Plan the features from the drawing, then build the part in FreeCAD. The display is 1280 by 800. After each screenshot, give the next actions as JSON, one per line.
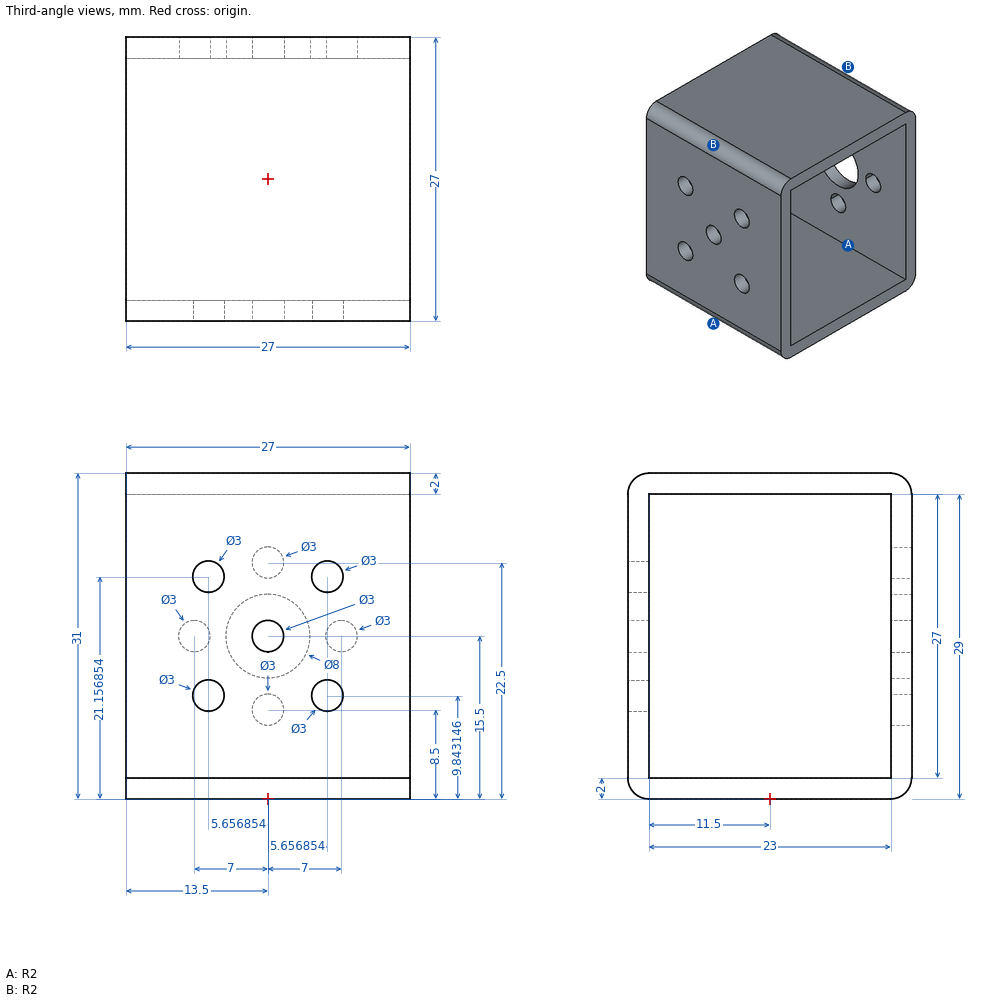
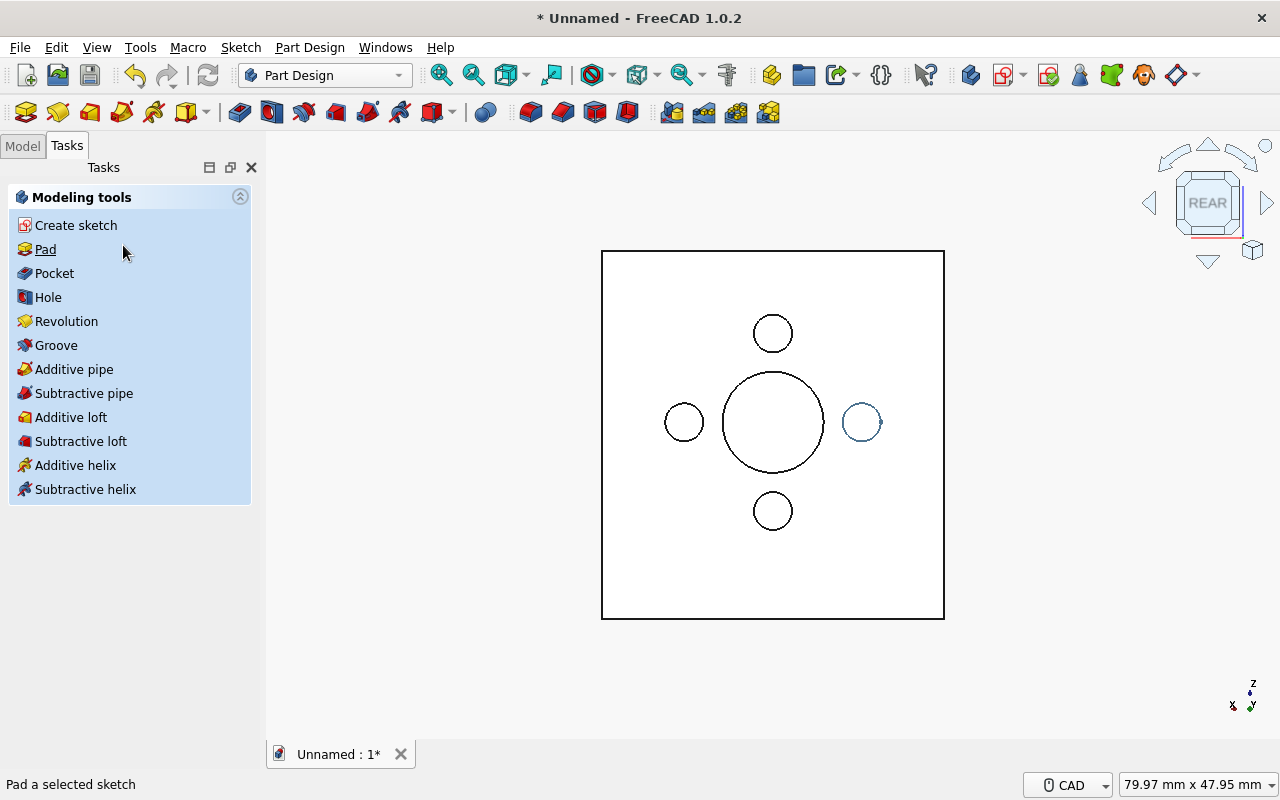
{"action": "left_click", "coordinate": [240, 112]}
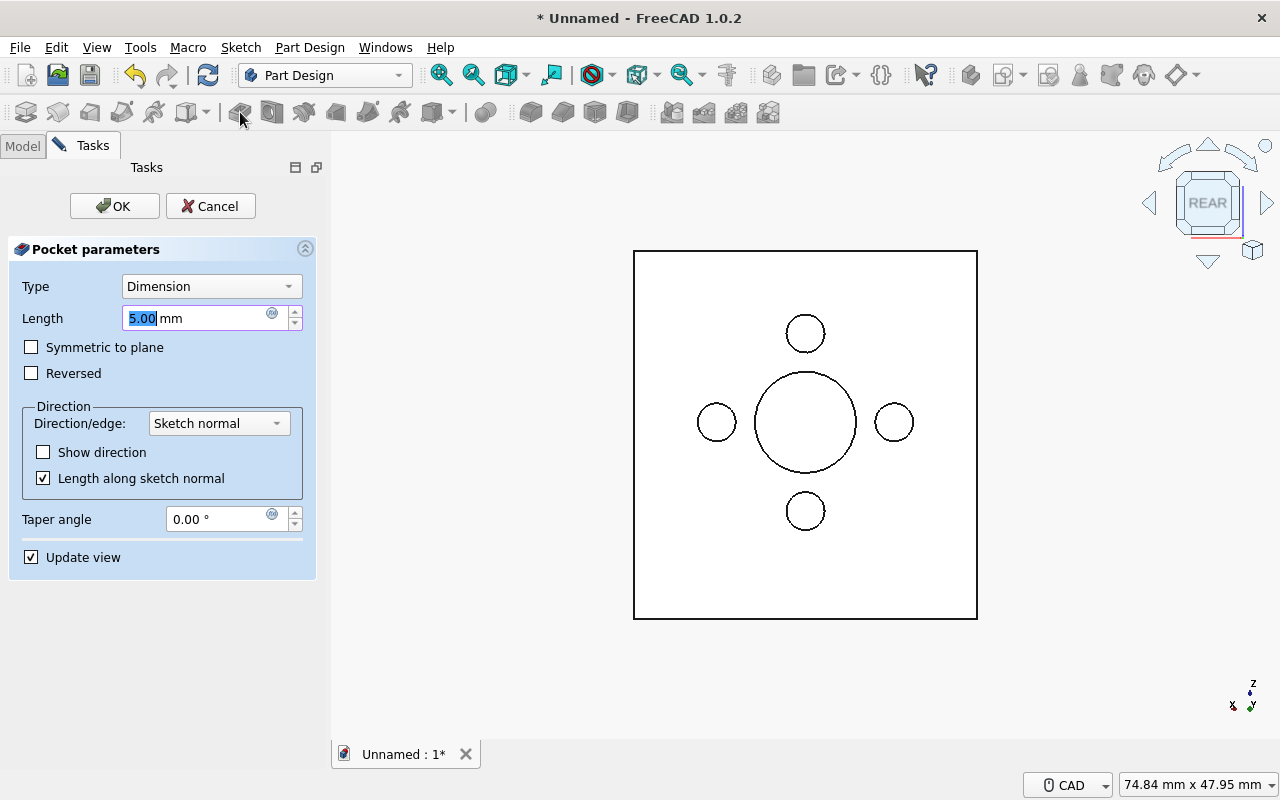
{"action": "left_click", "coordinate": [212, 286]}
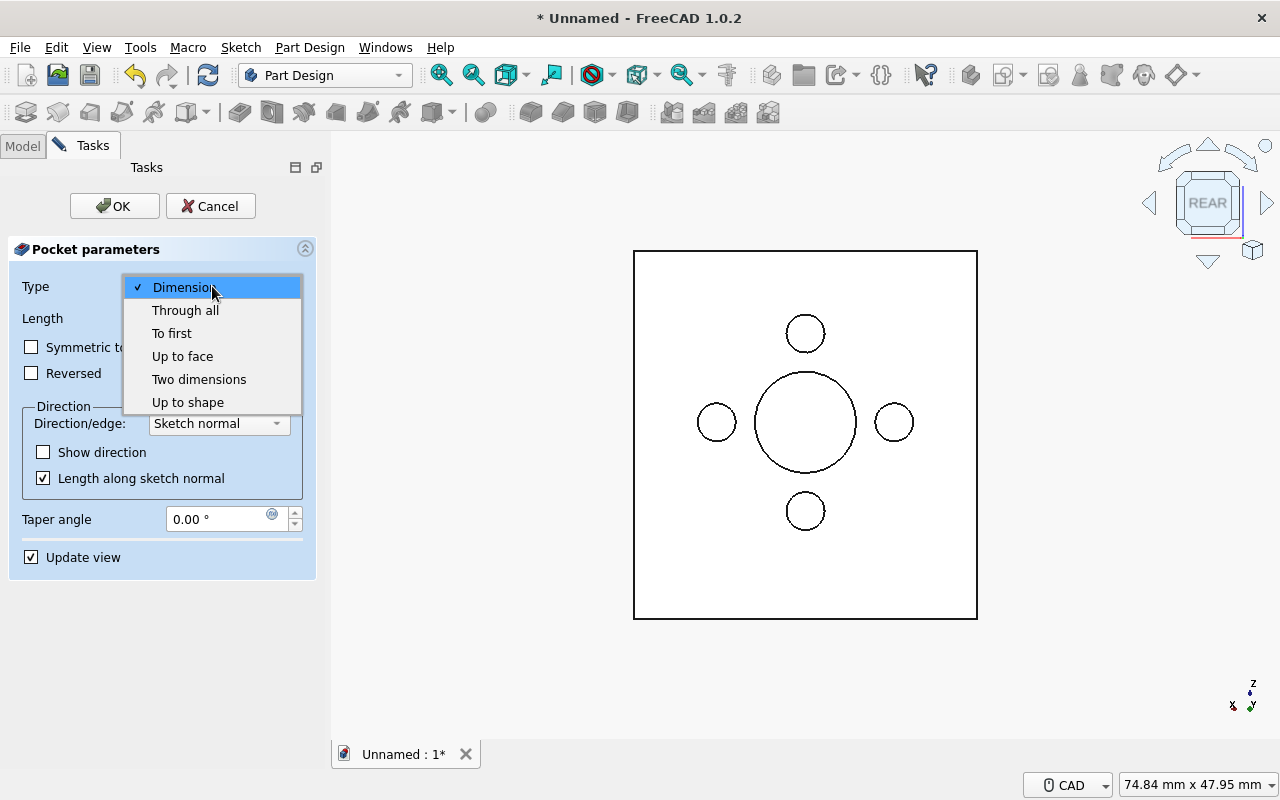
{"action": "left_click", "coordinate": [212, 334]}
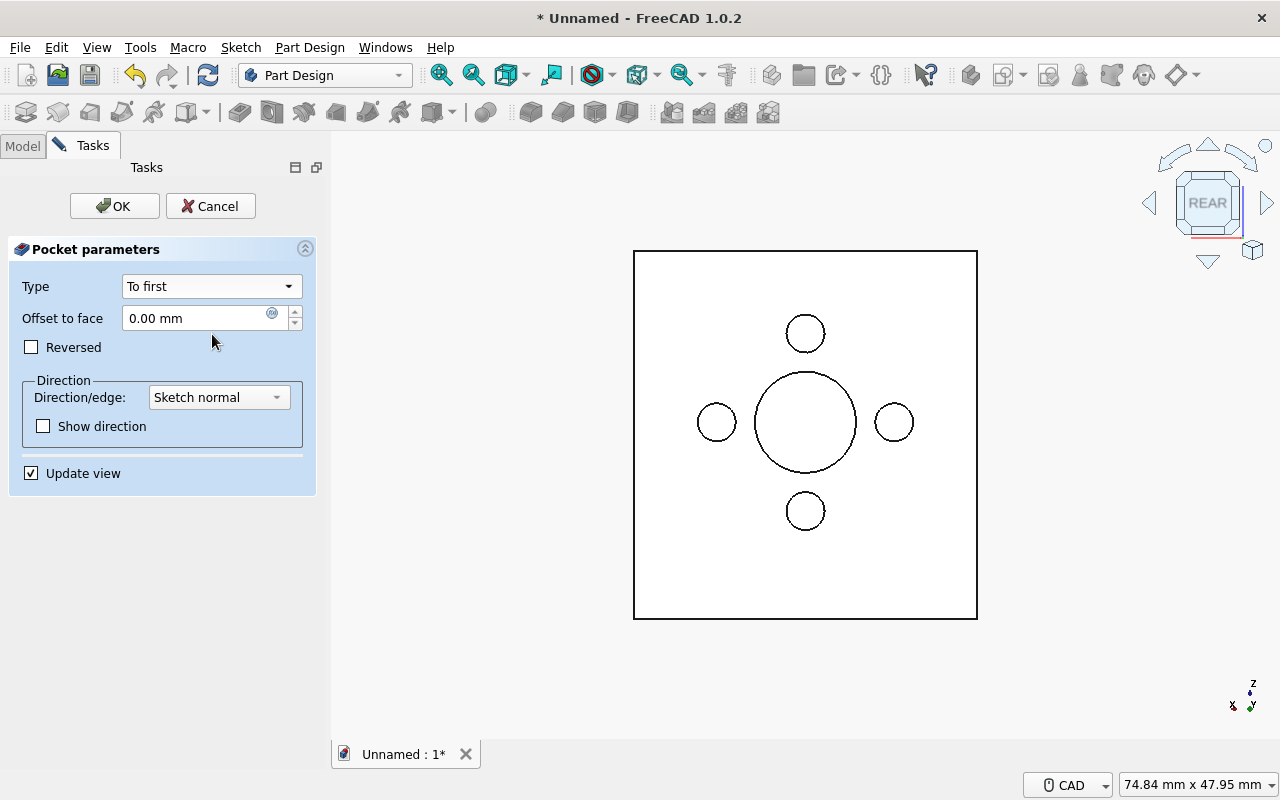
{"action": "left_click", "coordinate": [115, 206]}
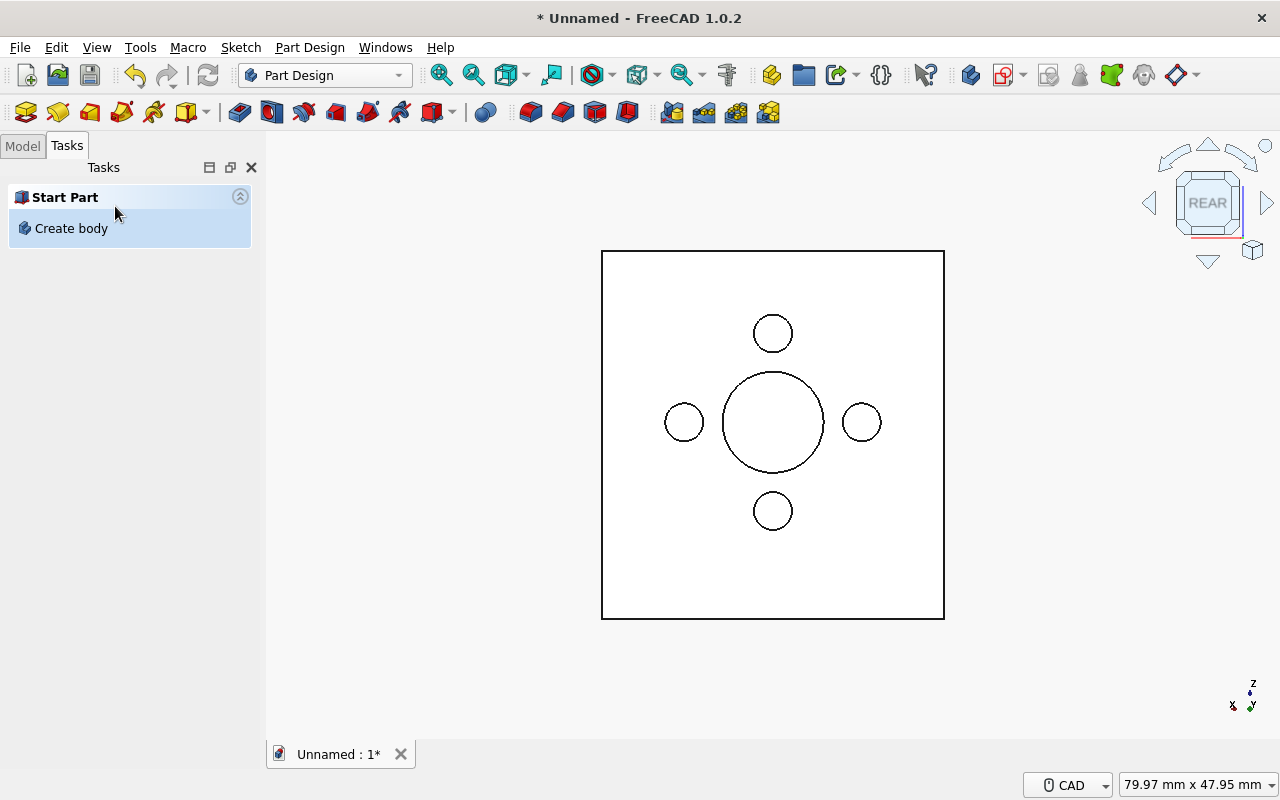
{"action": "key", "text": "0"}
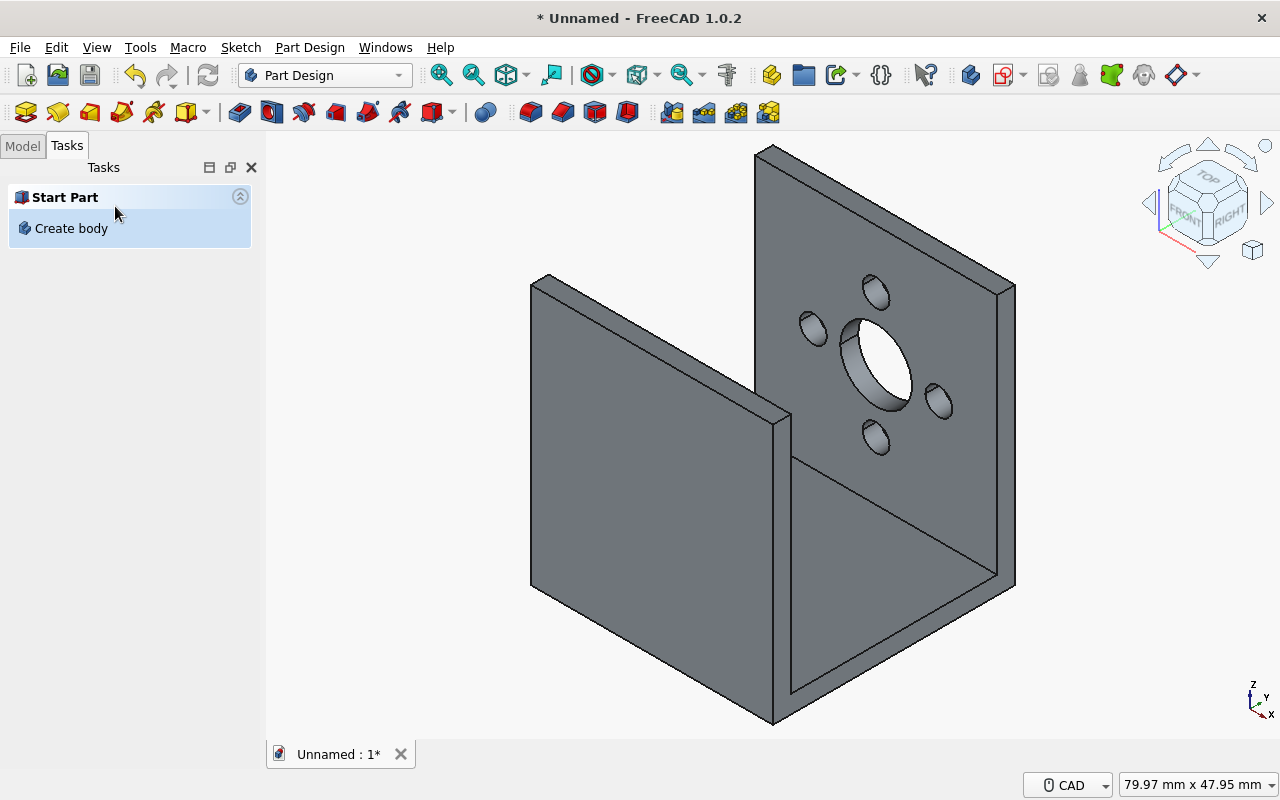
{"action": "left_click", "coordinate": [652, 504]}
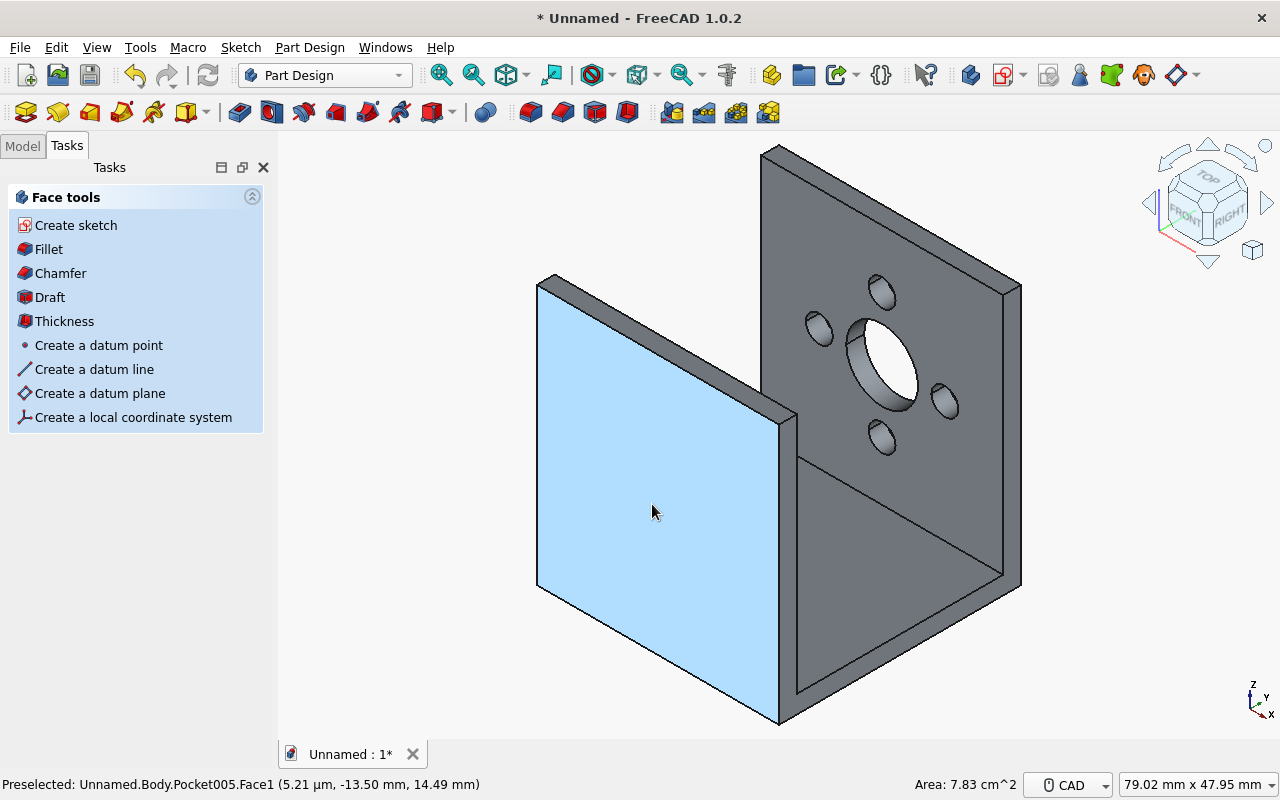
{"action": "left_click", "coordinate": [1004, 76]}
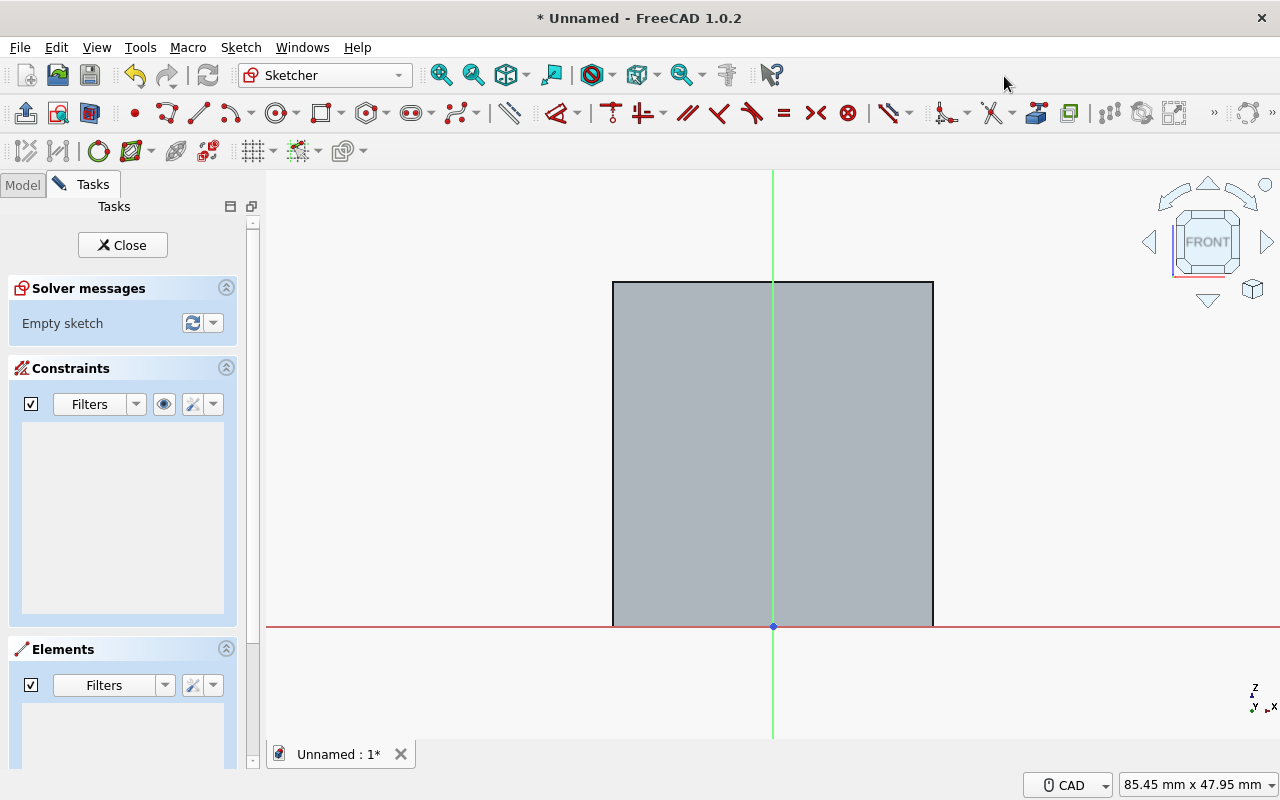
{"action": "scroll", "coordinate": [780, 441], "scroll_direction": "up", "scroll_amount": 12}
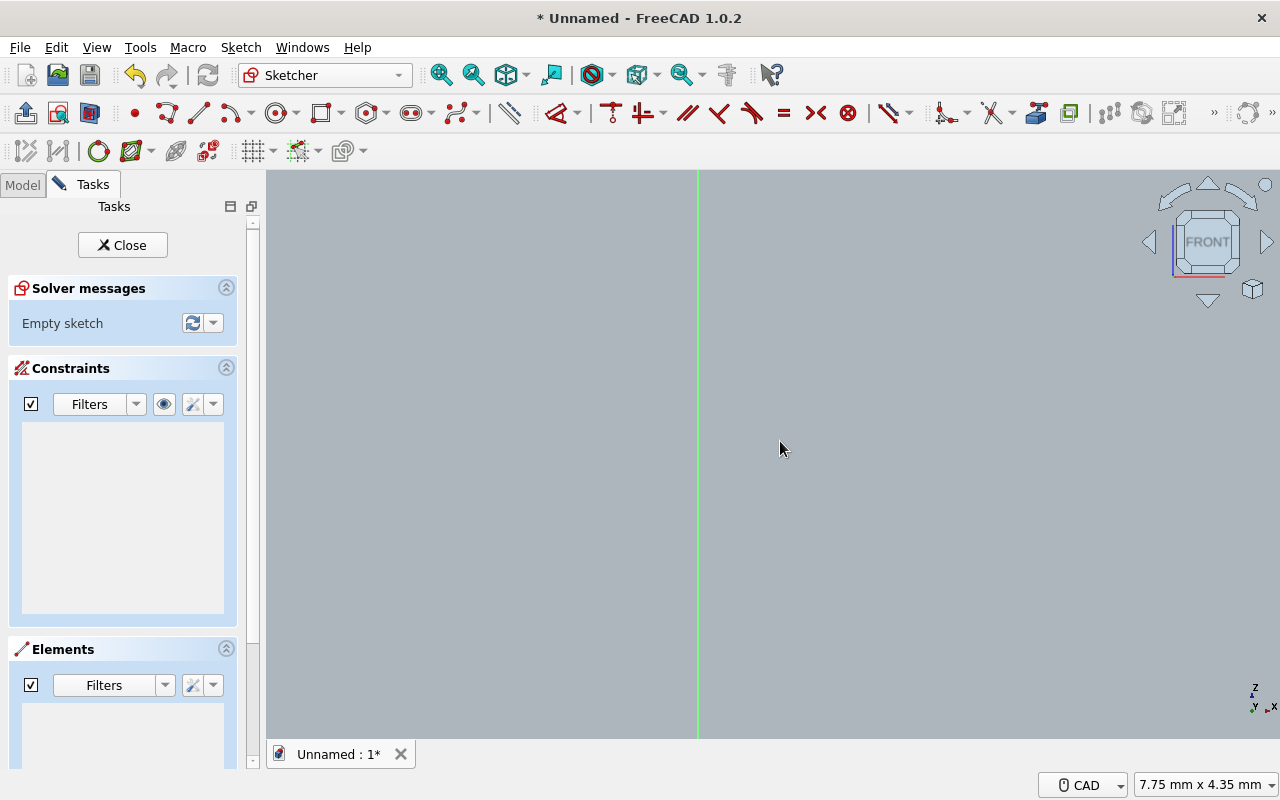
{"action": "left_click", "coordinate": [276, 114]}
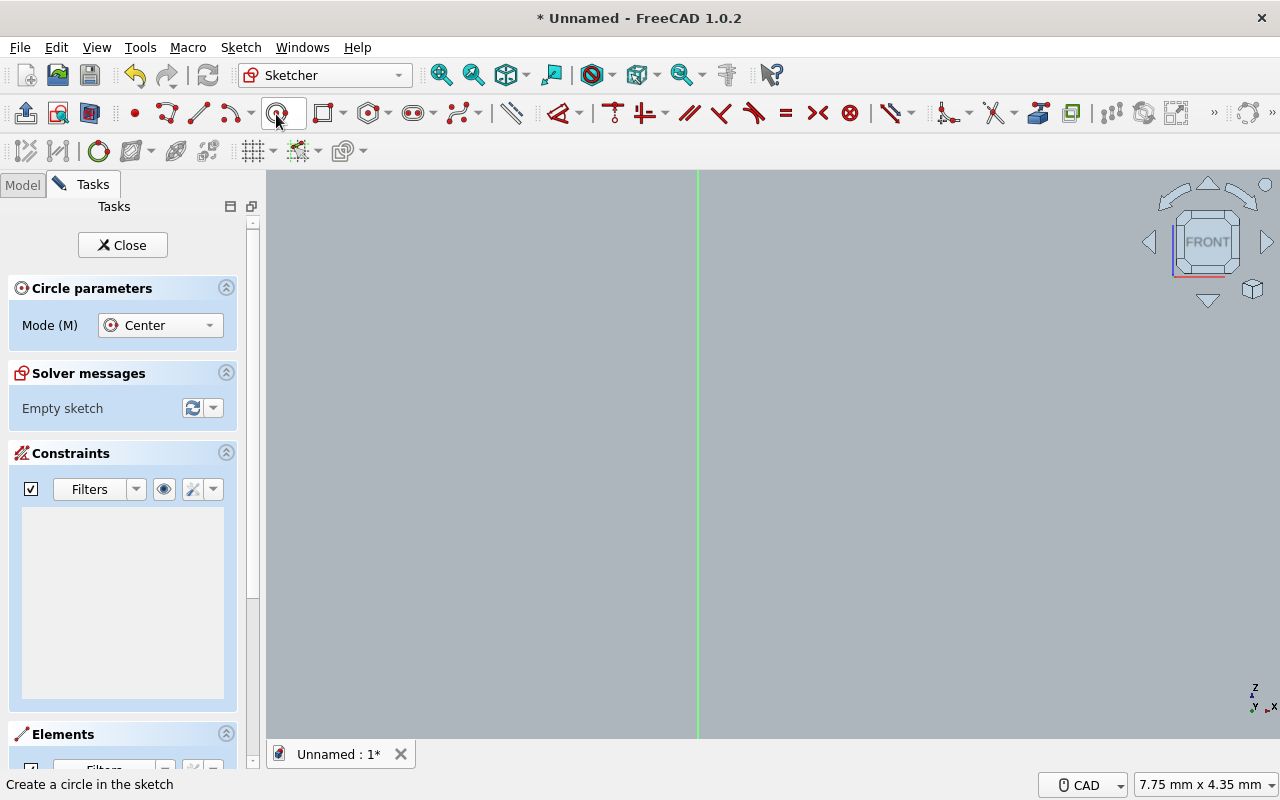
{"action": "left_click", "coordinate": [698, 454]}
{"action": "mouse_move", "coordinate": [836, 315]}